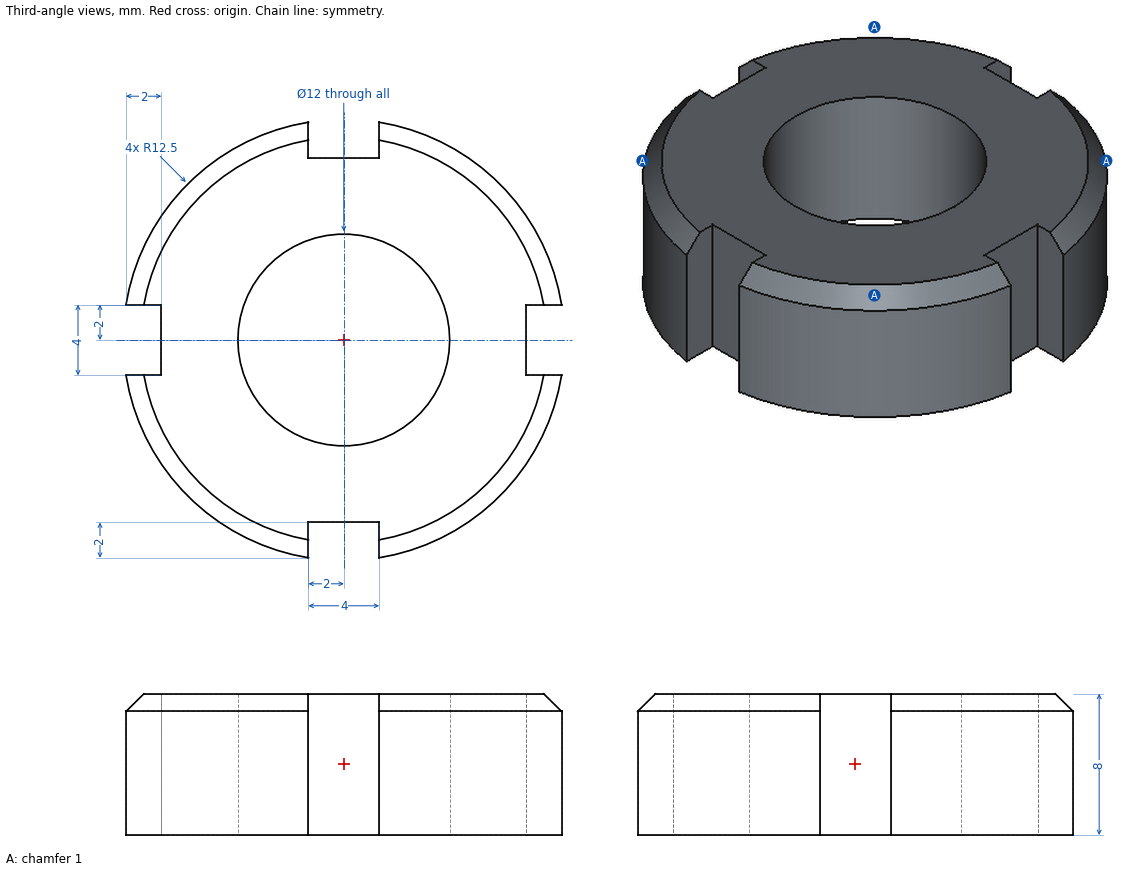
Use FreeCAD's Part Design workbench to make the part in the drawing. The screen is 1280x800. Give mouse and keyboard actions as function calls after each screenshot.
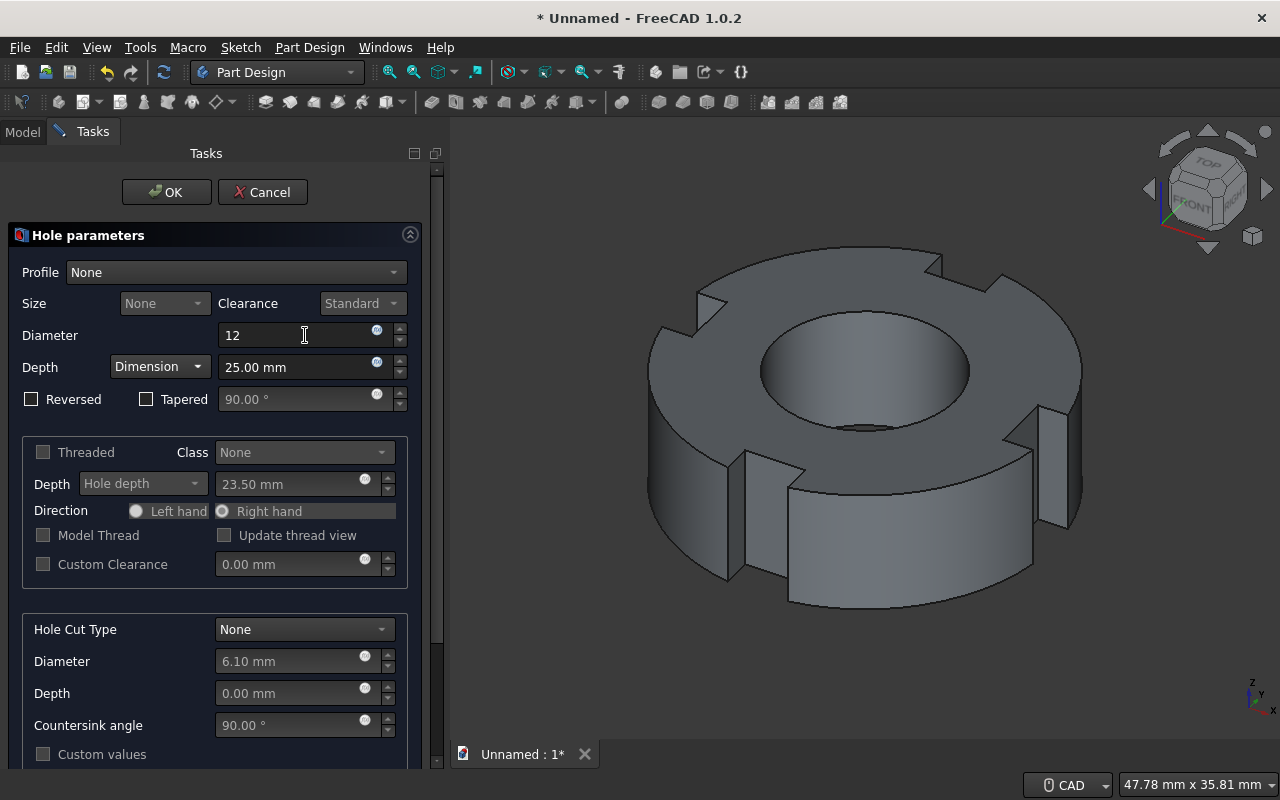
click(161, 366)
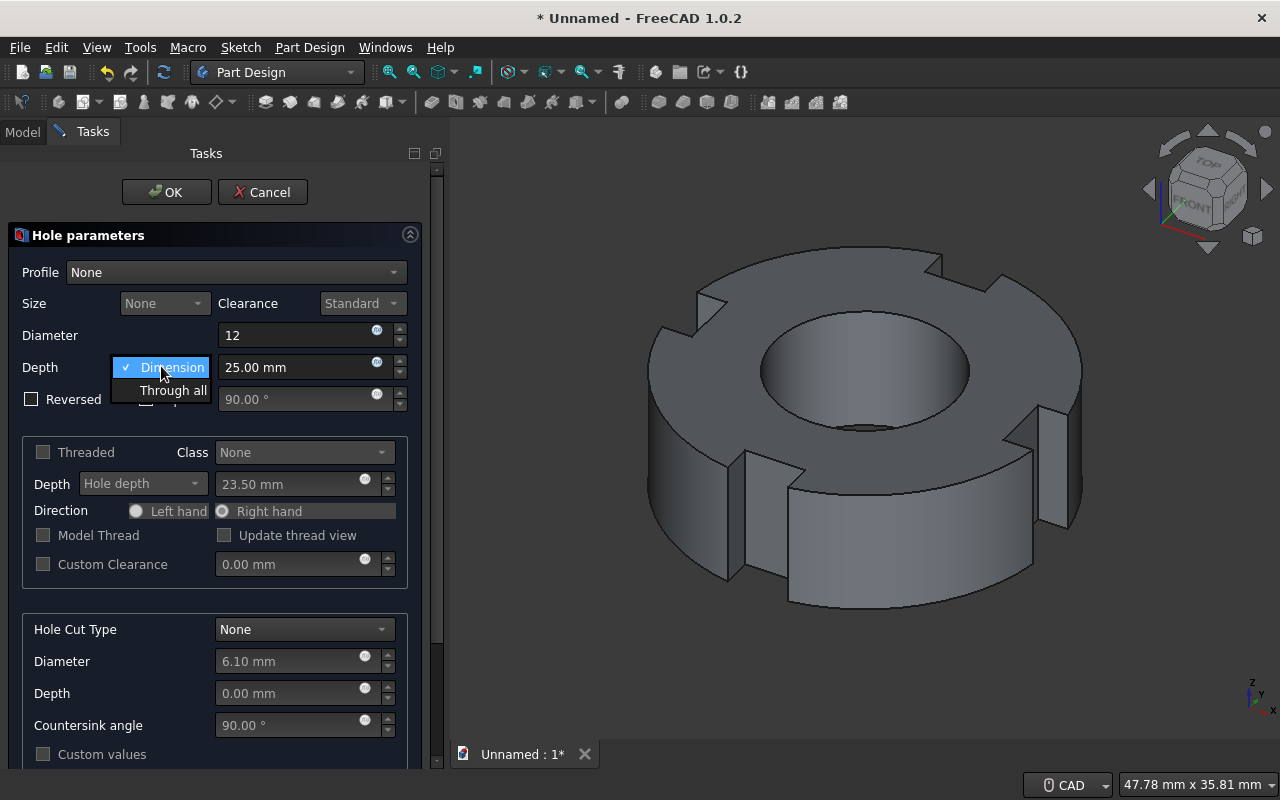
click(160, 390)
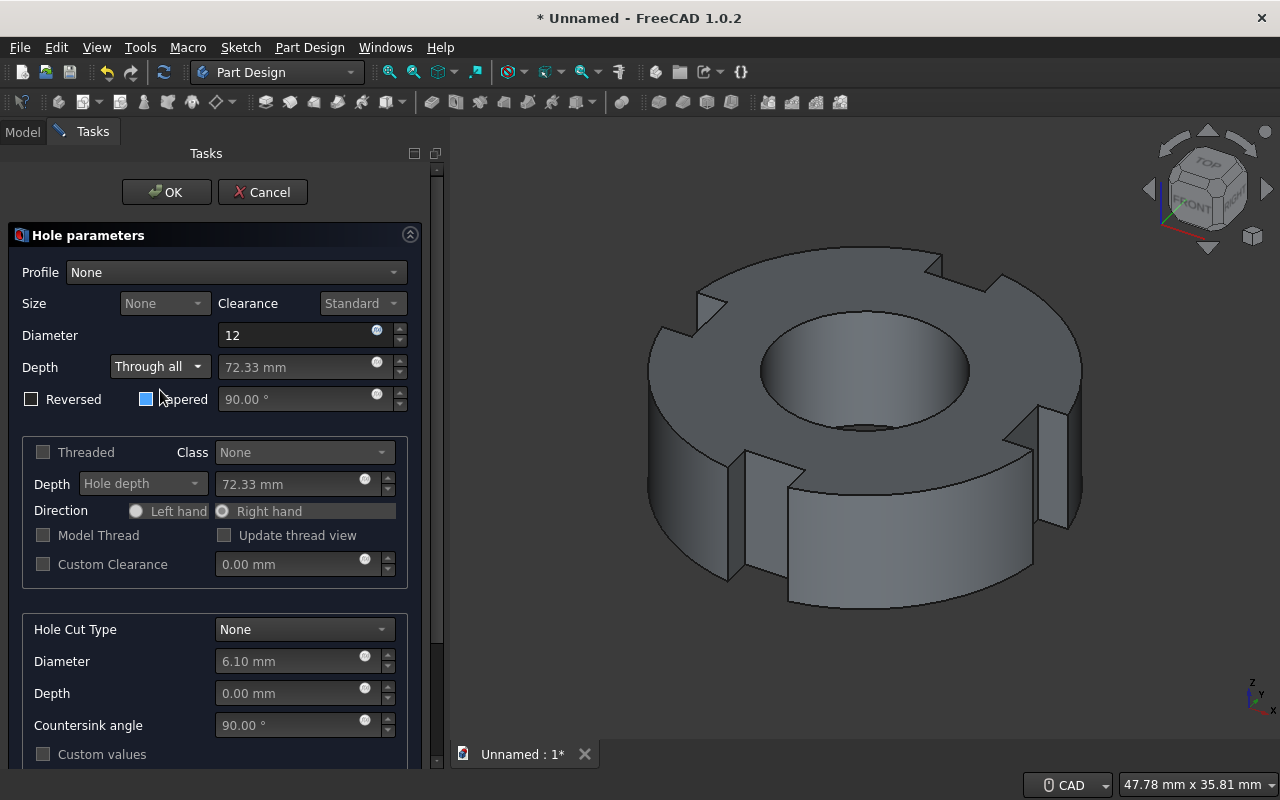
click(167, 192)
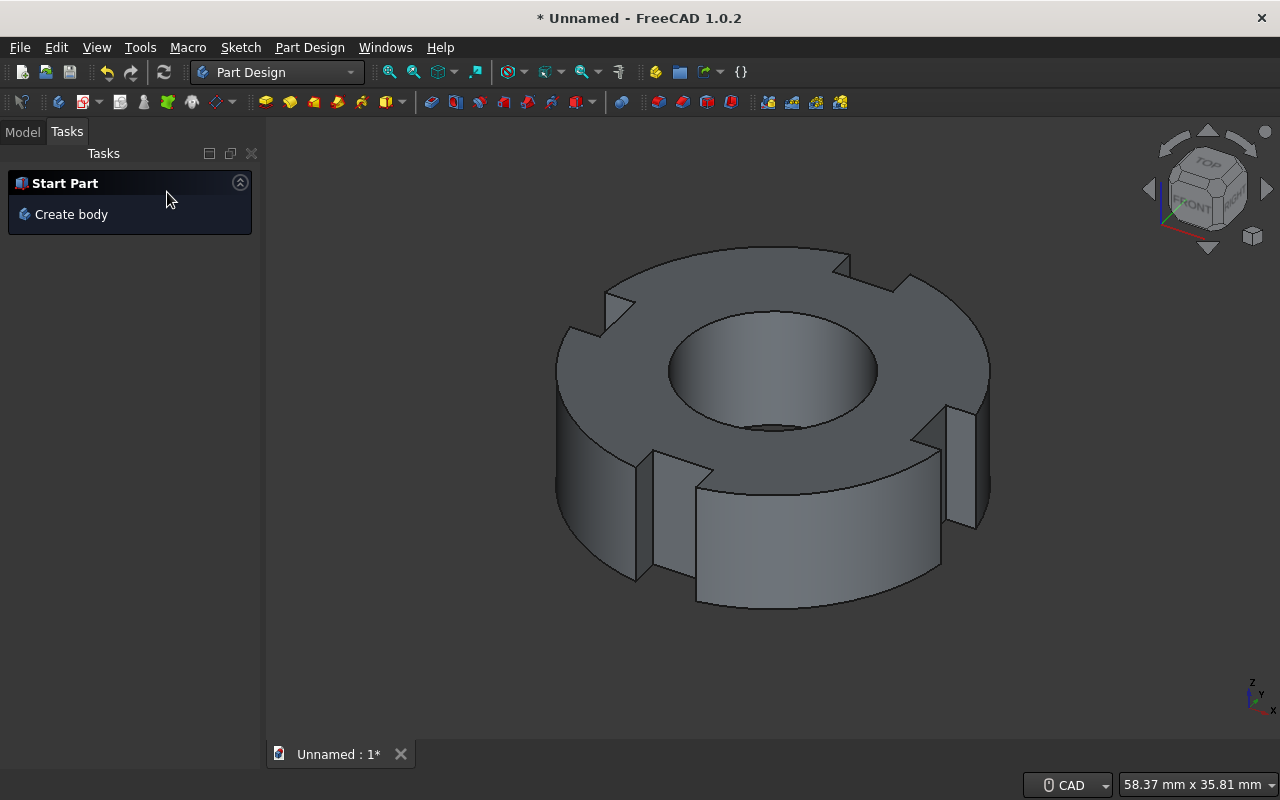
click(563, 402)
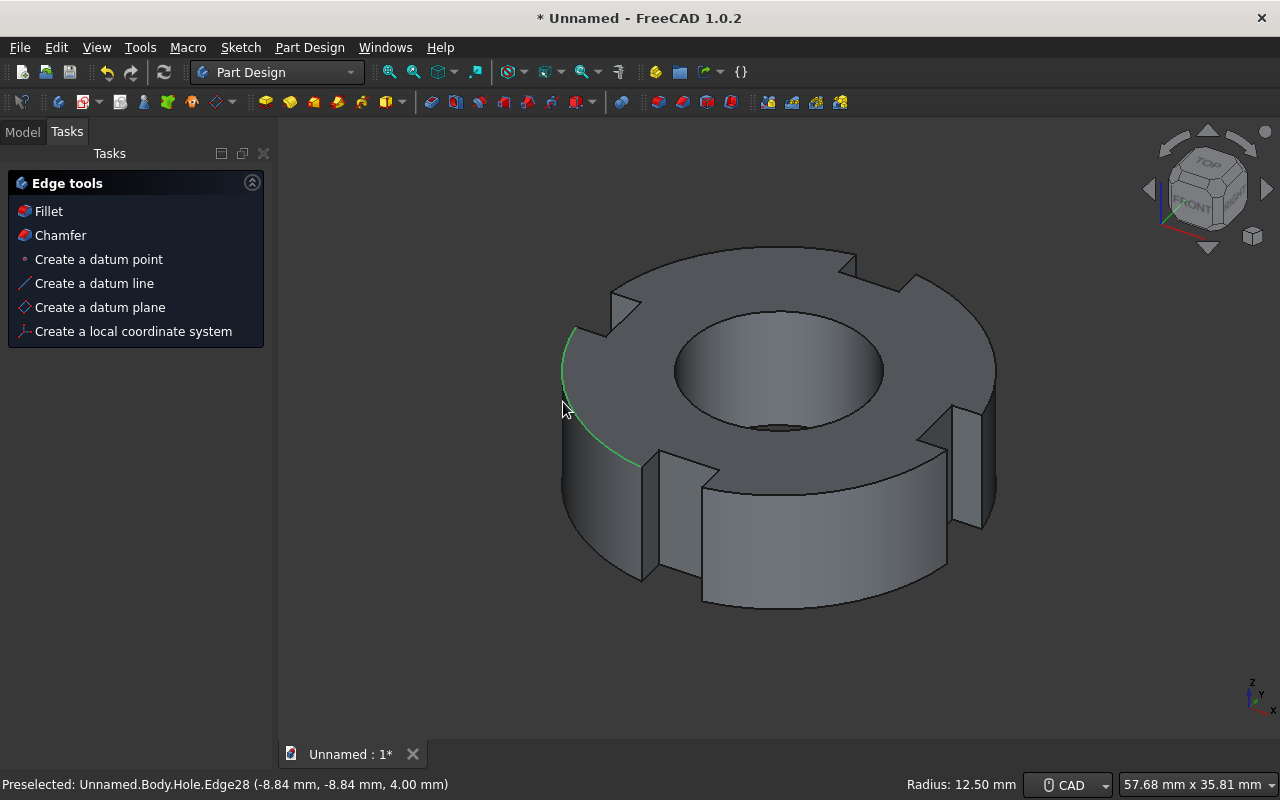
click(835, 490, ctrl)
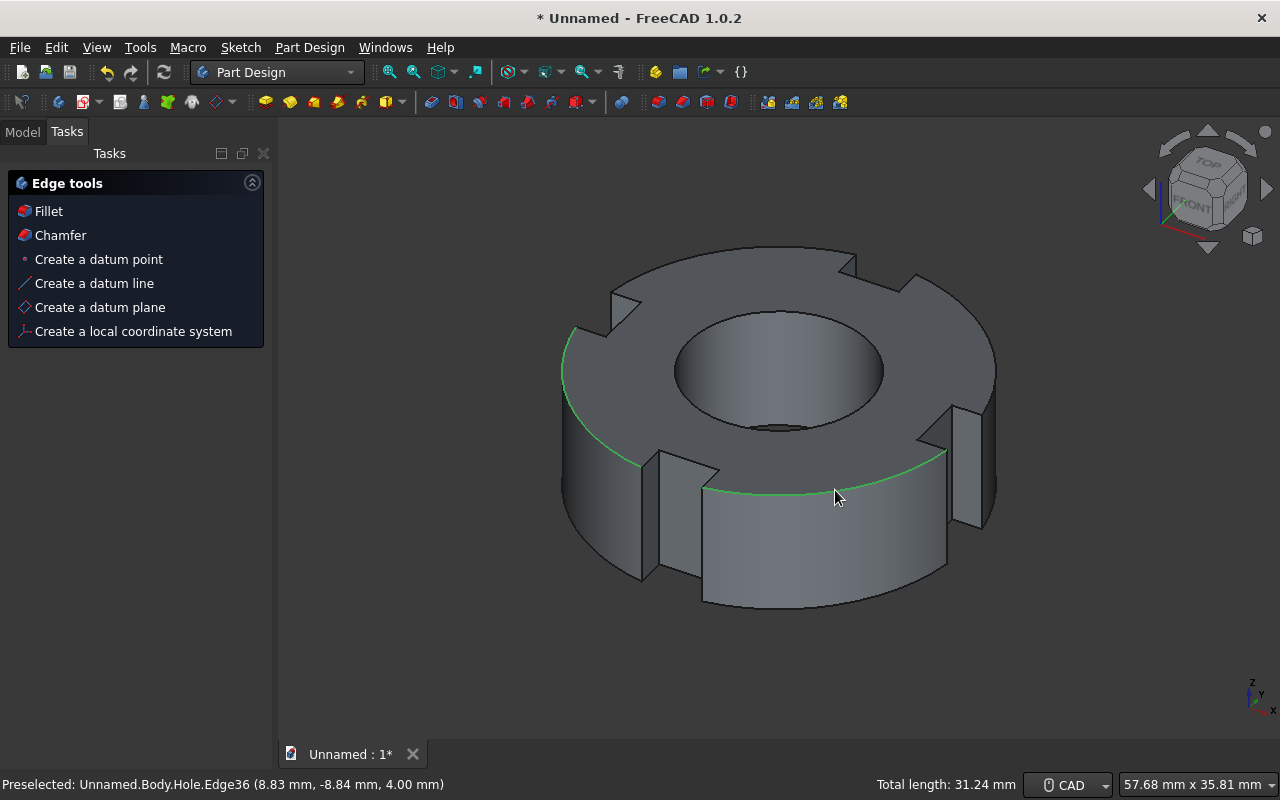
click(995, 384, ctrl)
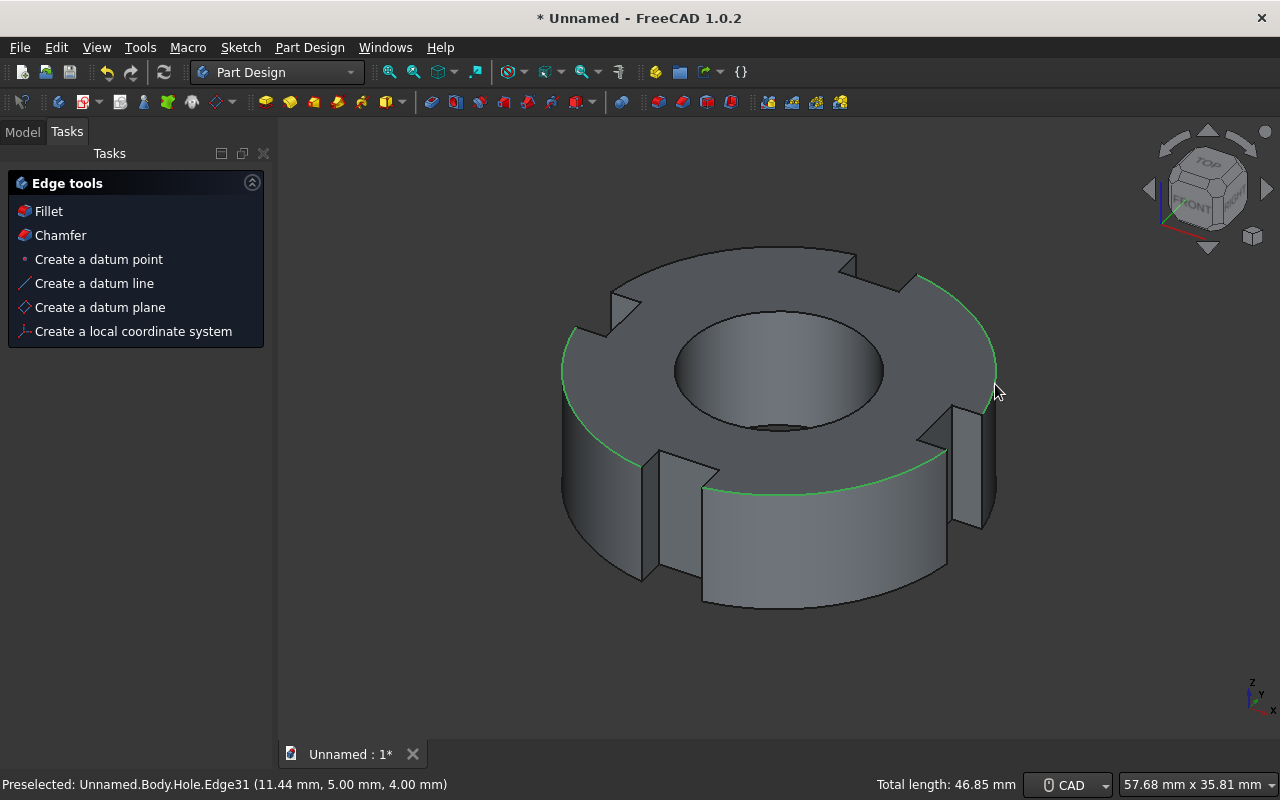
key(0)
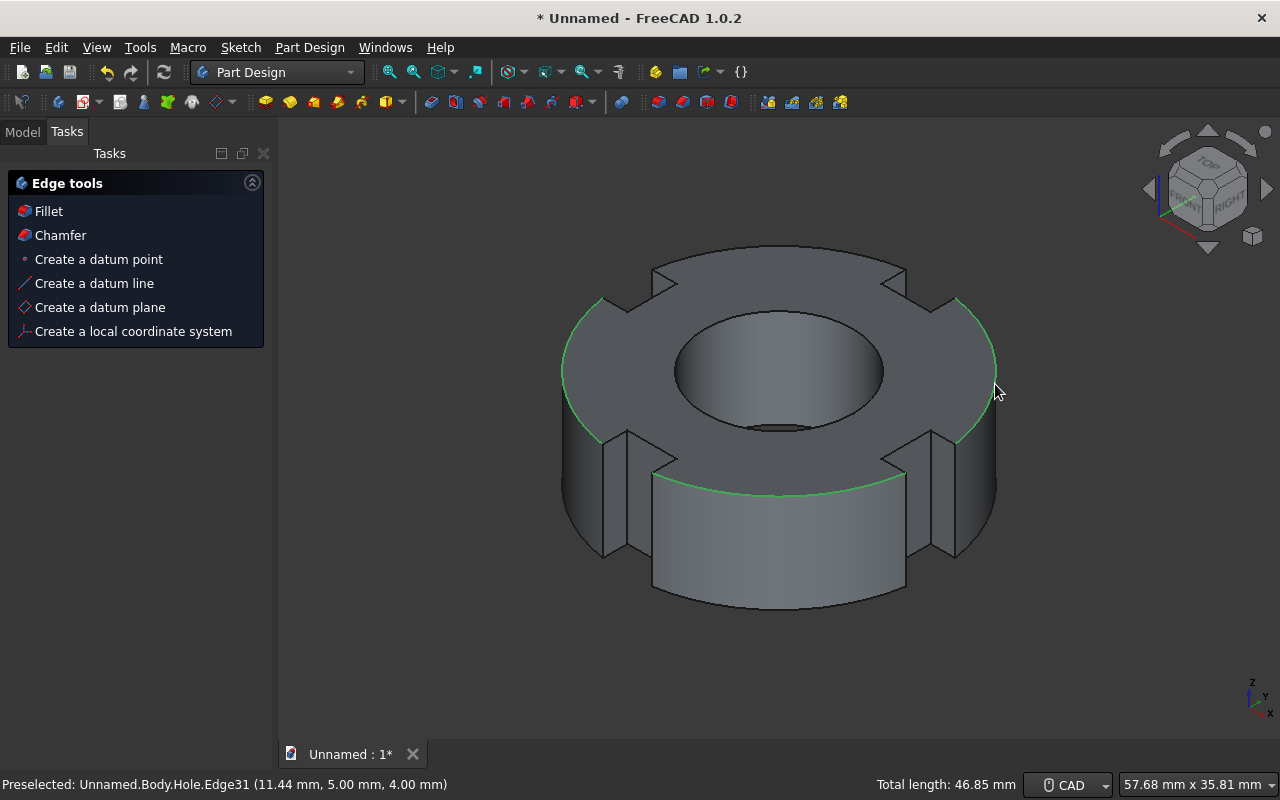
key(2)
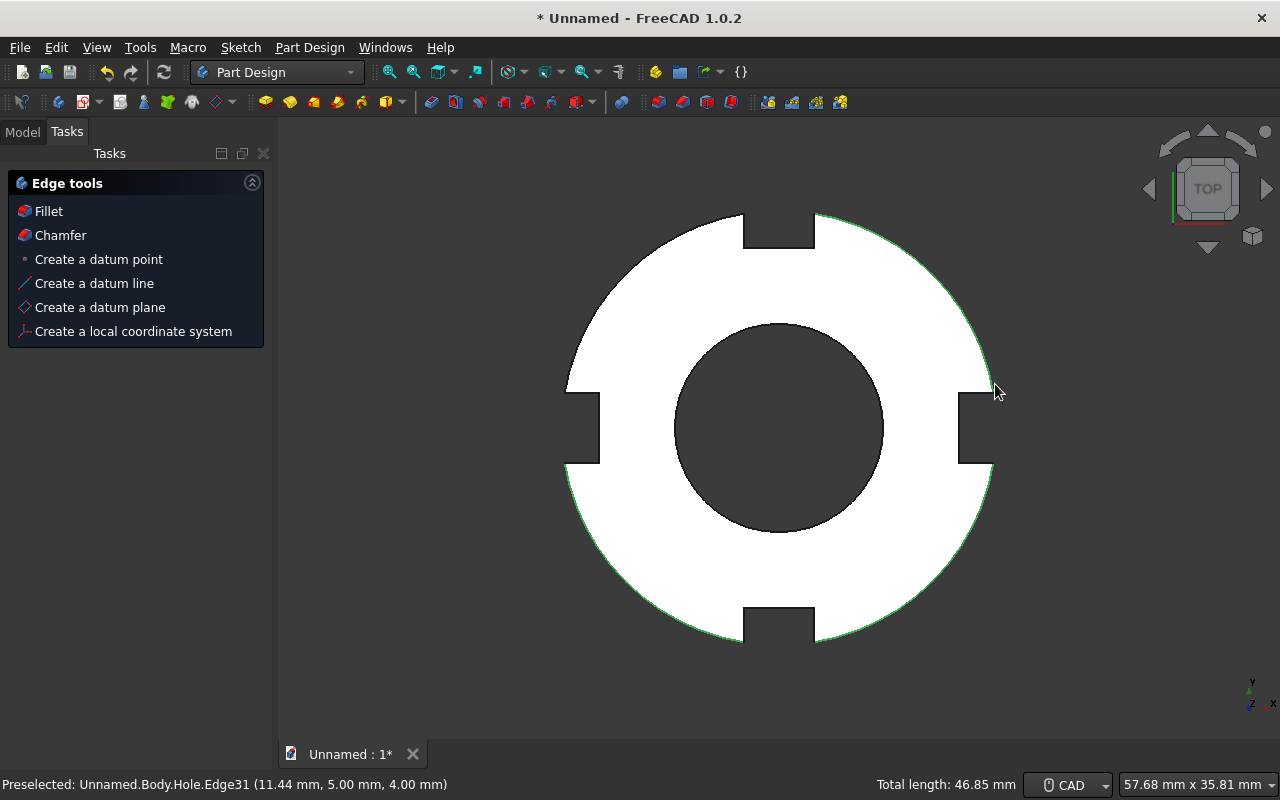
click(625, 273, ctrl)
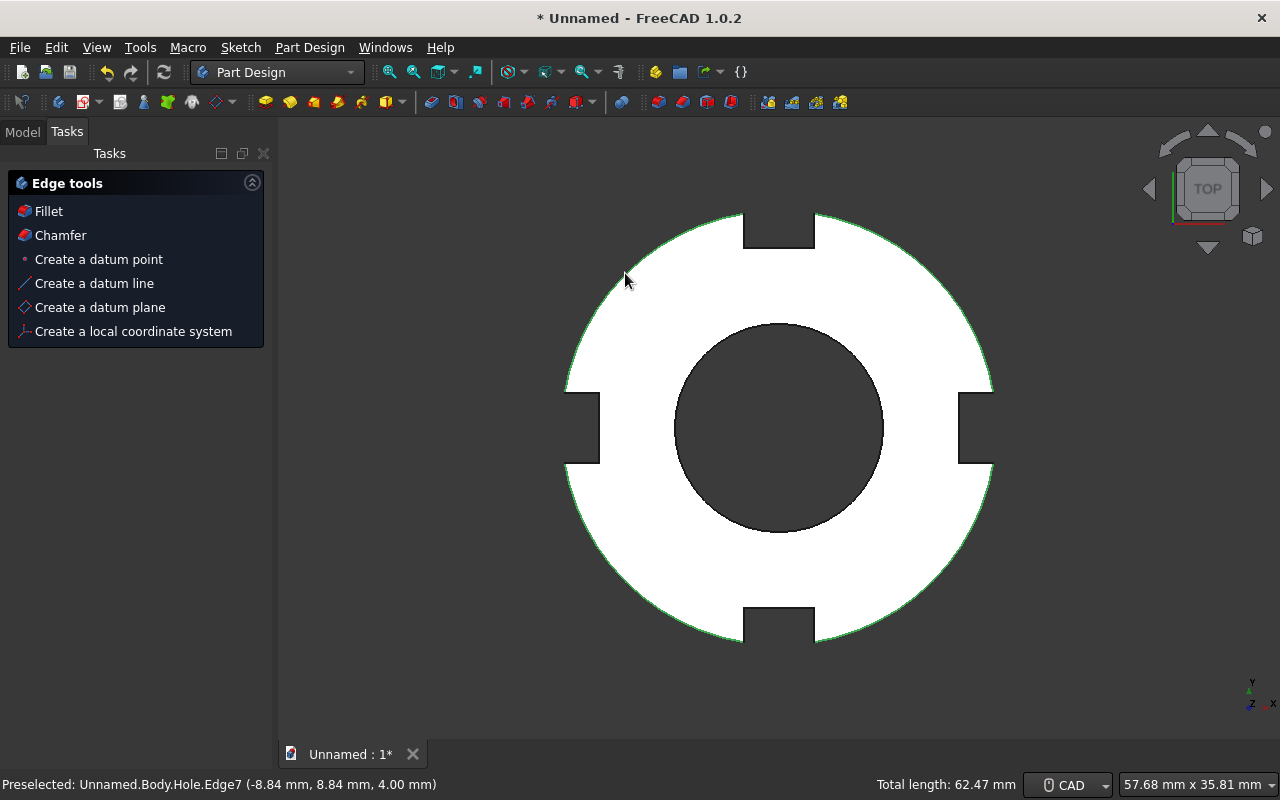
click(684, 102)